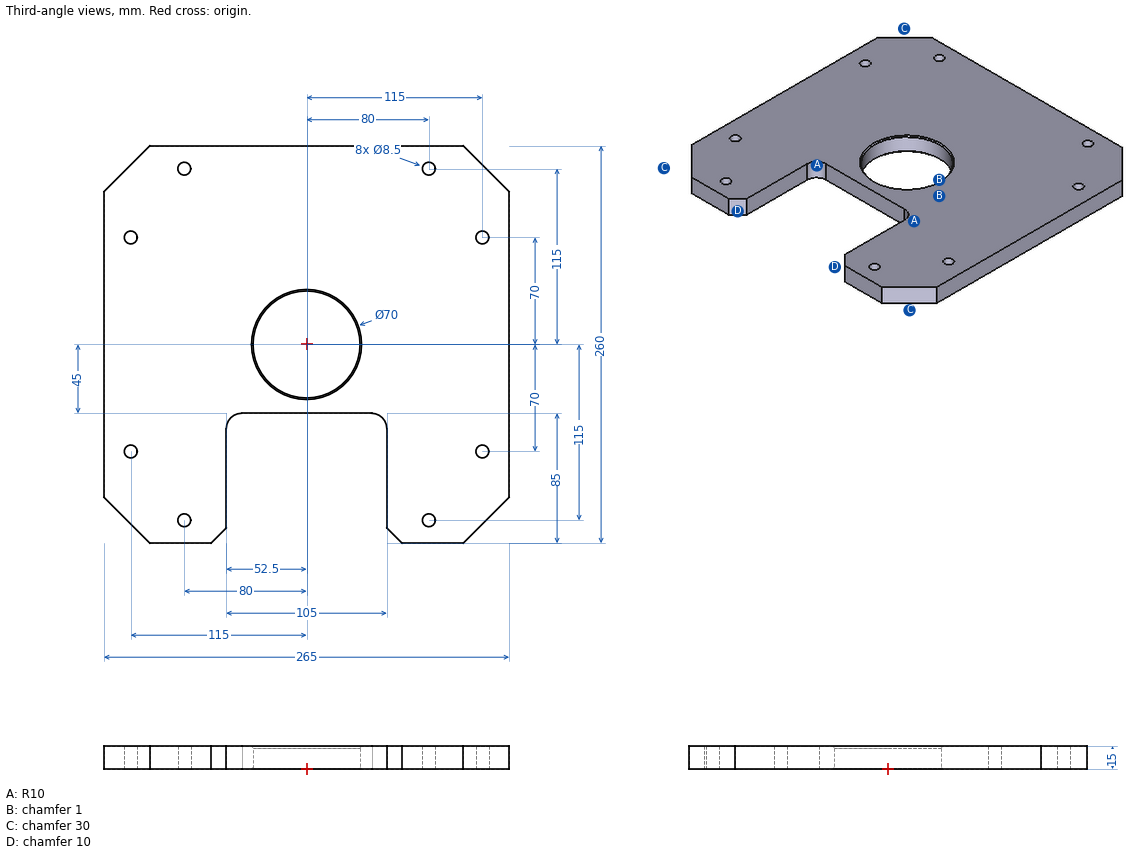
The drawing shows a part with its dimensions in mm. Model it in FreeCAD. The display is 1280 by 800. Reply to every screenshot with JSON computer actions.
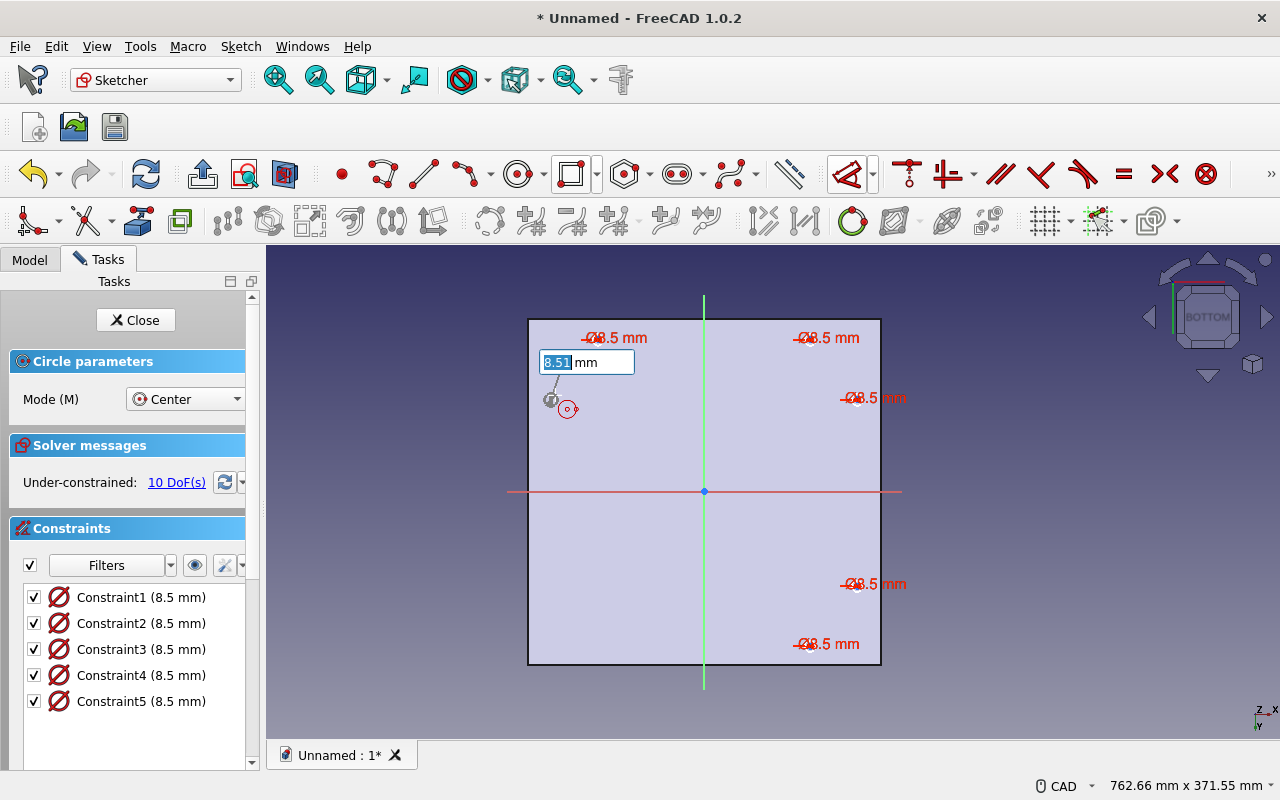
{"action": "type", "text": "8.5"}
{"action": "key", "text": "Return"}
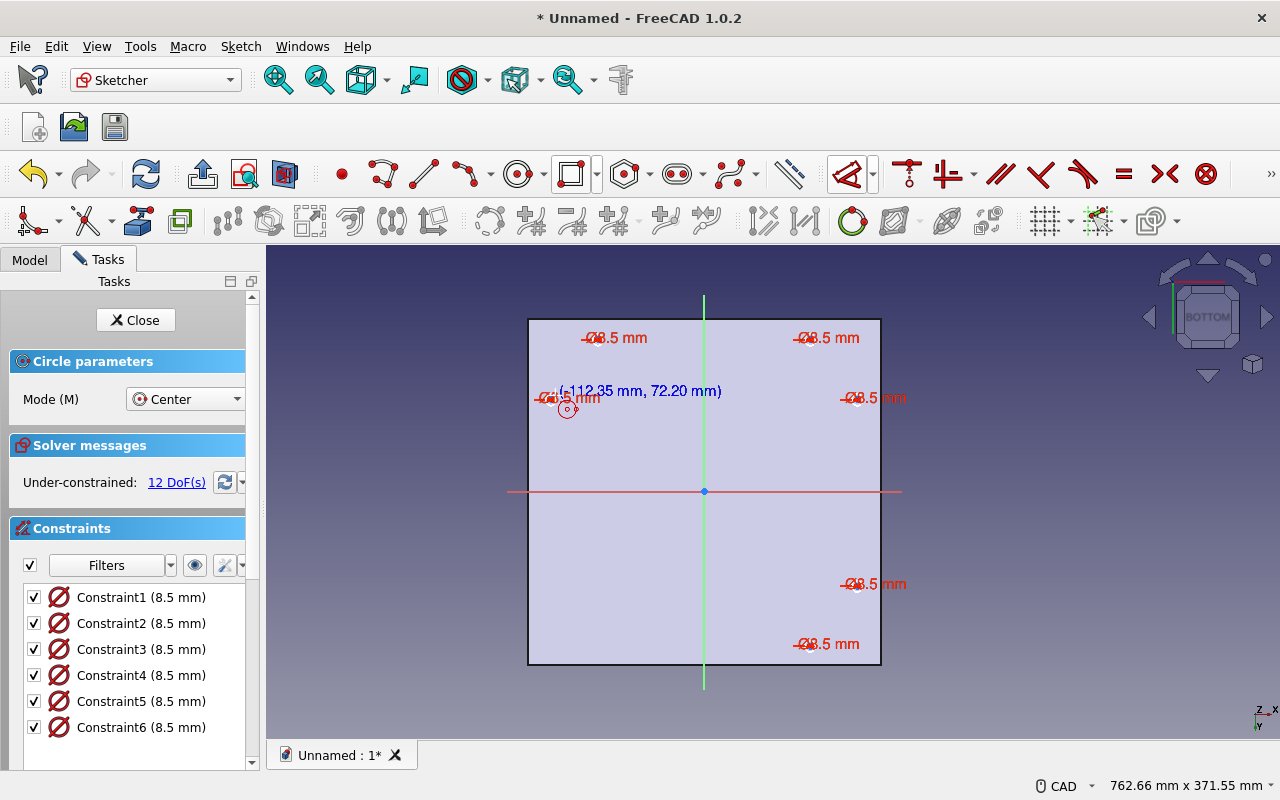
{"action": "scroll", "coordinate": [551, 585], "scroll_direction": "up", "scroll_amount": 7}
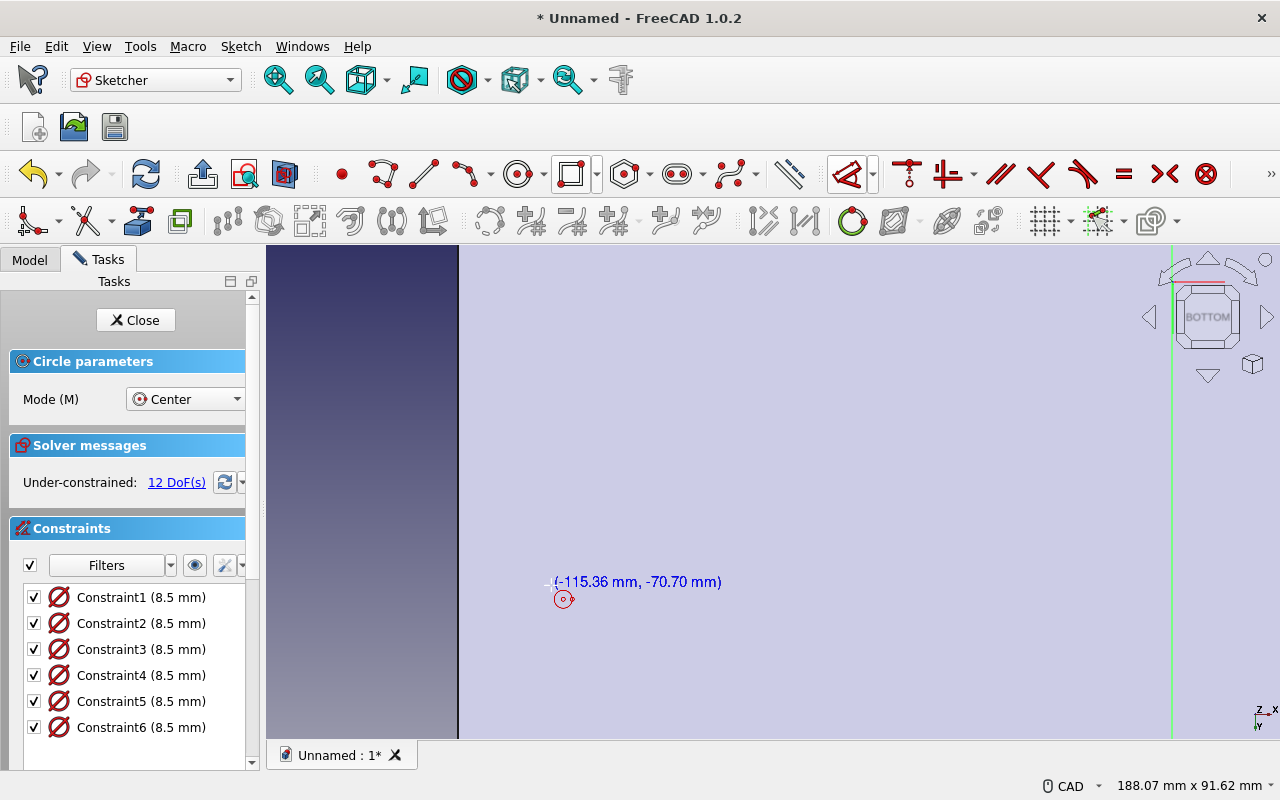
{"action": "scroll", "coordinate": [551, 586], "scroll_direction": "down", "scroll_amount": 7}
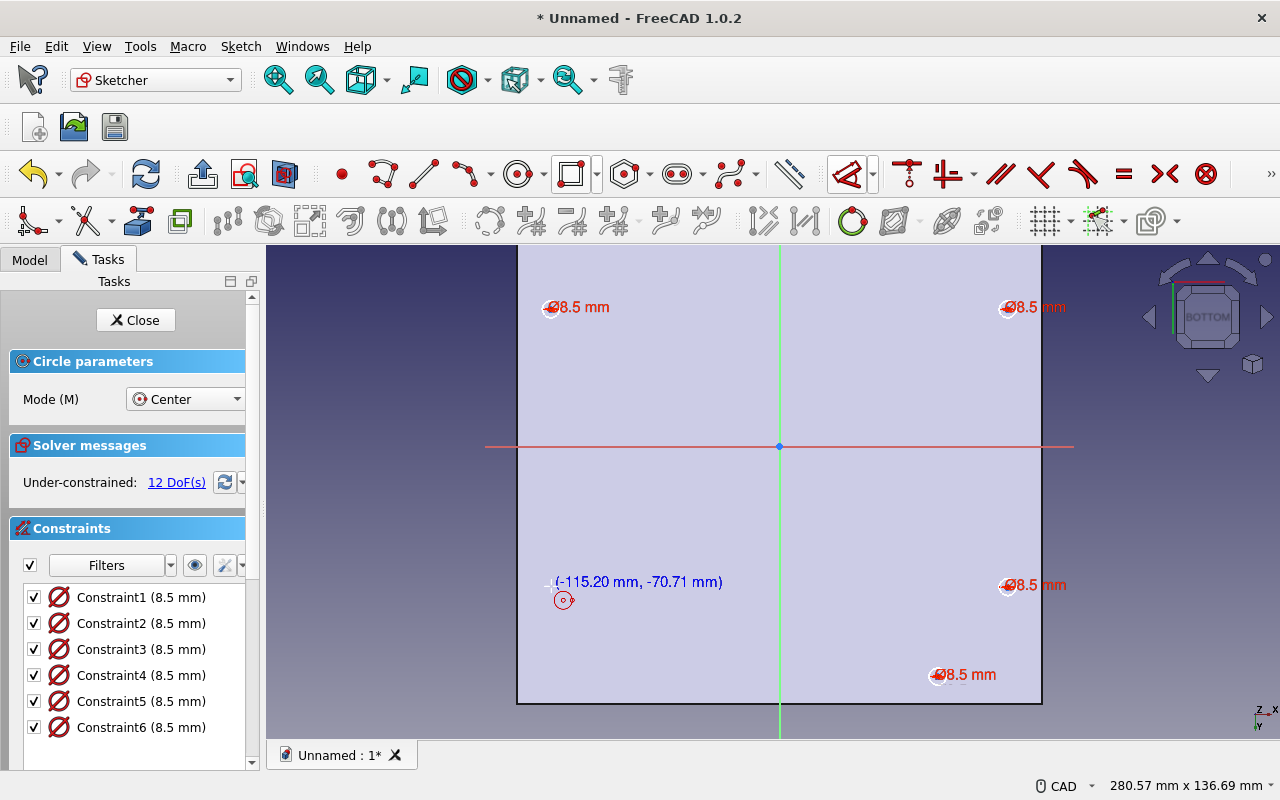
{"action": "left_click", "coordinate": [551, 586]}
{"action": "mouse_move", "coordinate": [555, 582]}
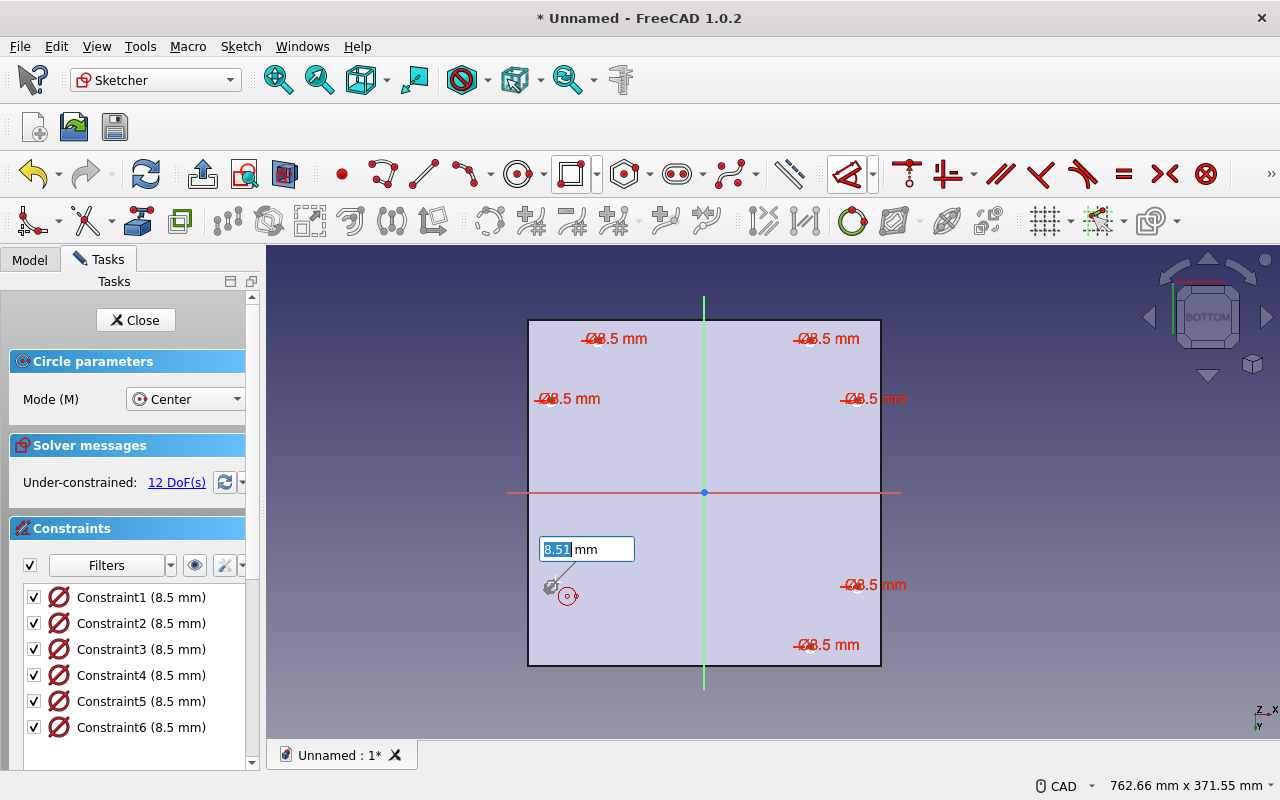
{"action": "type", "text": "8.5"}
{"action": "key", "text": "Return"}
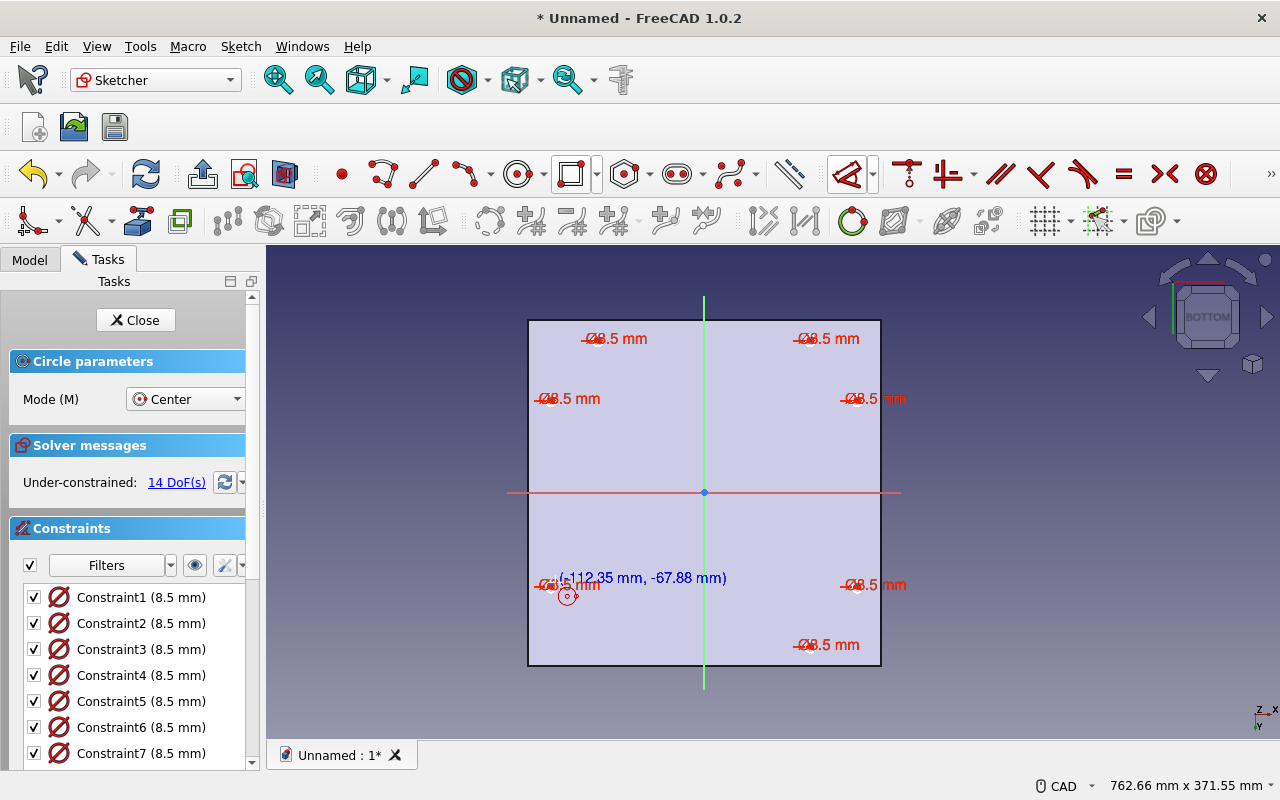
{"action": "scroll", "coordinate": [598, 646], "scroll_direction": "up", "scroll_amount": 7}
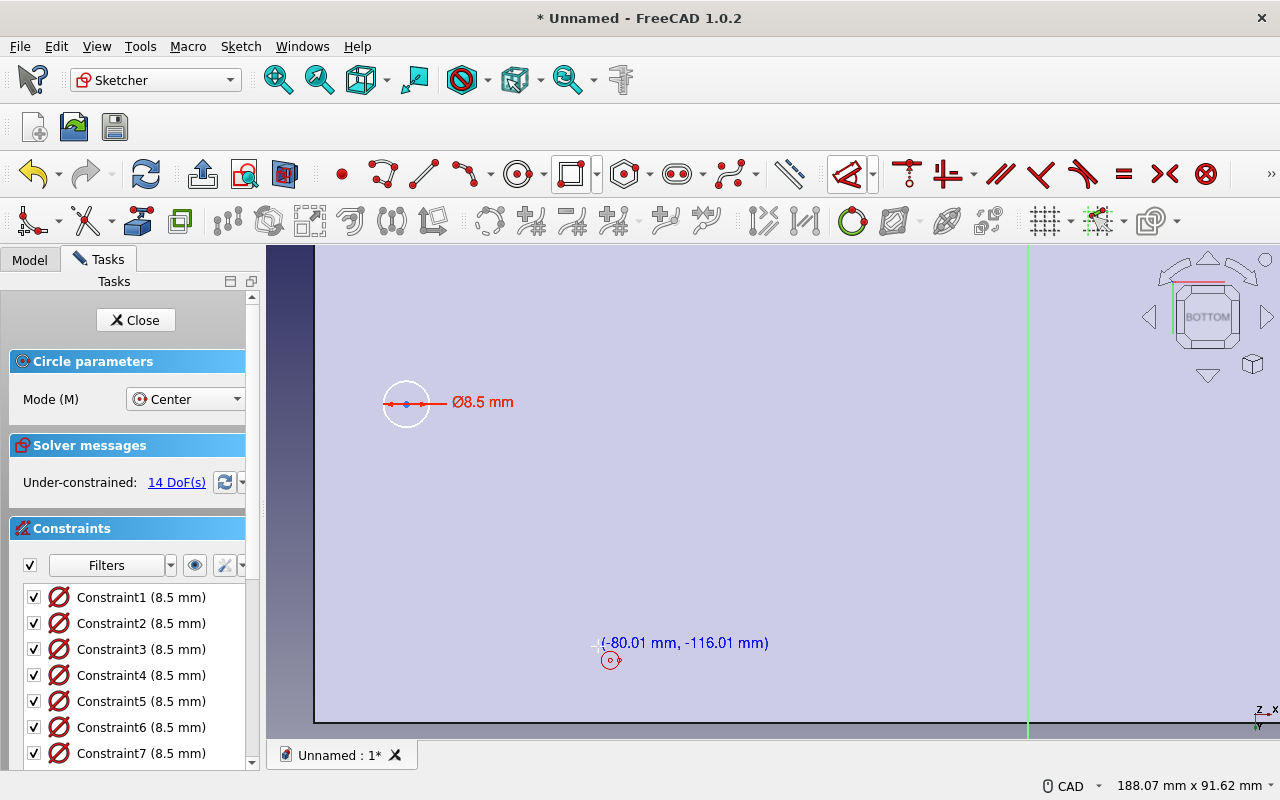
{"action": "scroll", "coordinate": [598, 646], "scroll_direction": "down", "scroll_amount": 7}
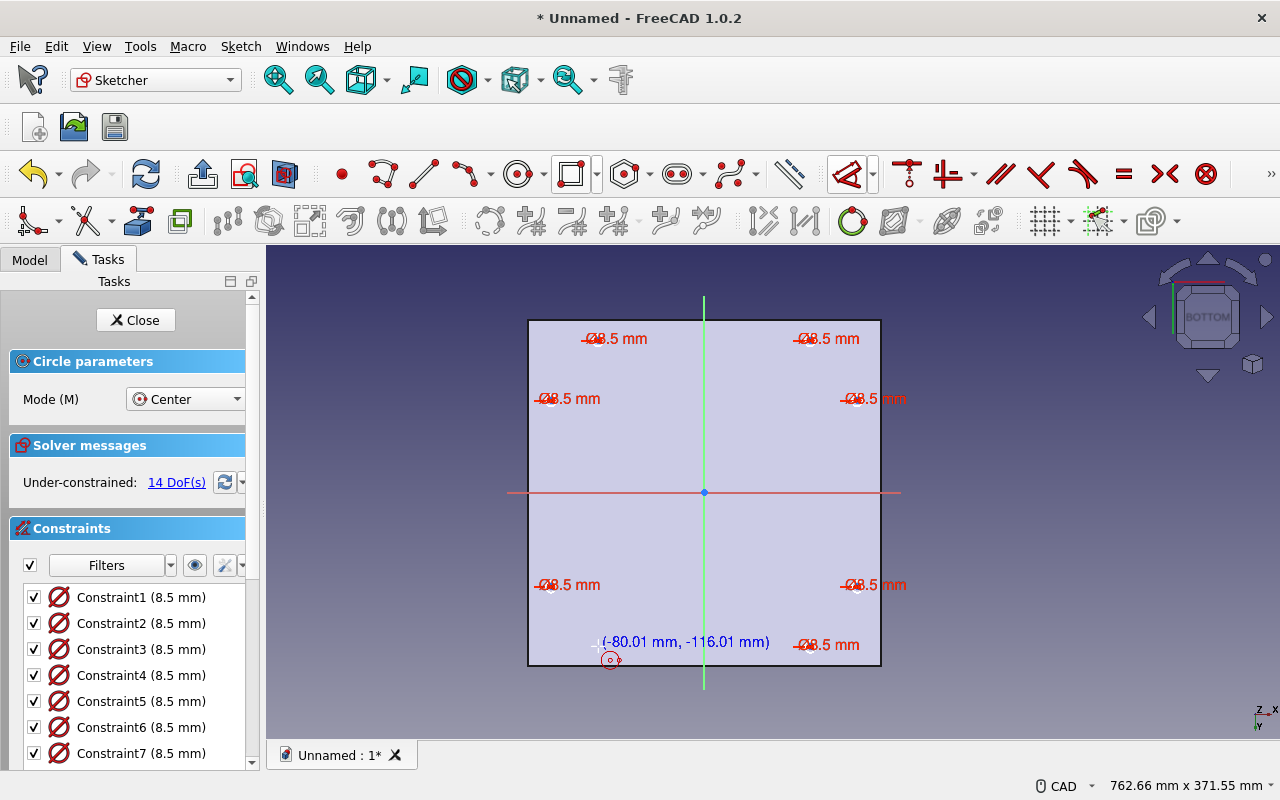
{"action": "left_click", "coordinate": [598, 646]}
{"action": "mouse_move", "coordinate": [602, 642]}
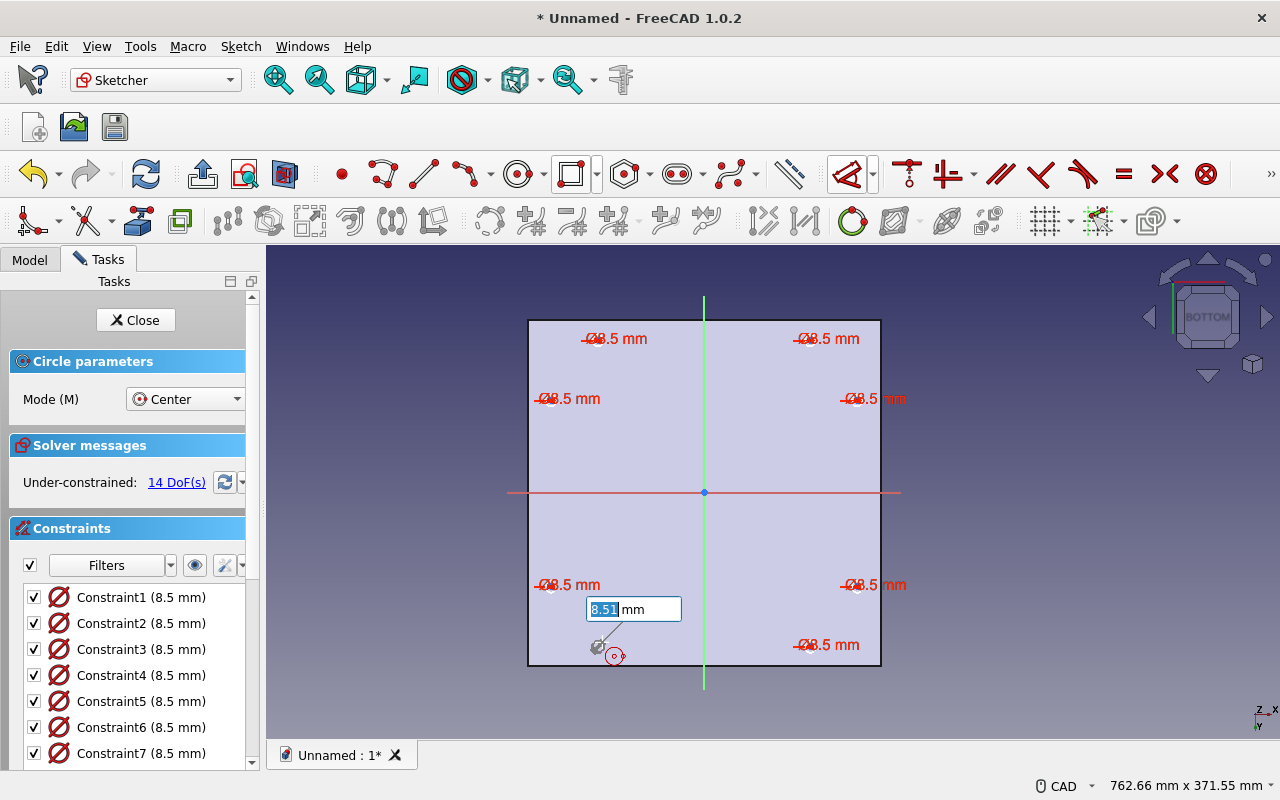
{"action": "type", "text": "8.5"}
{"action": "key", "text": "Return"}
{"action": "key", "text": "Escape"}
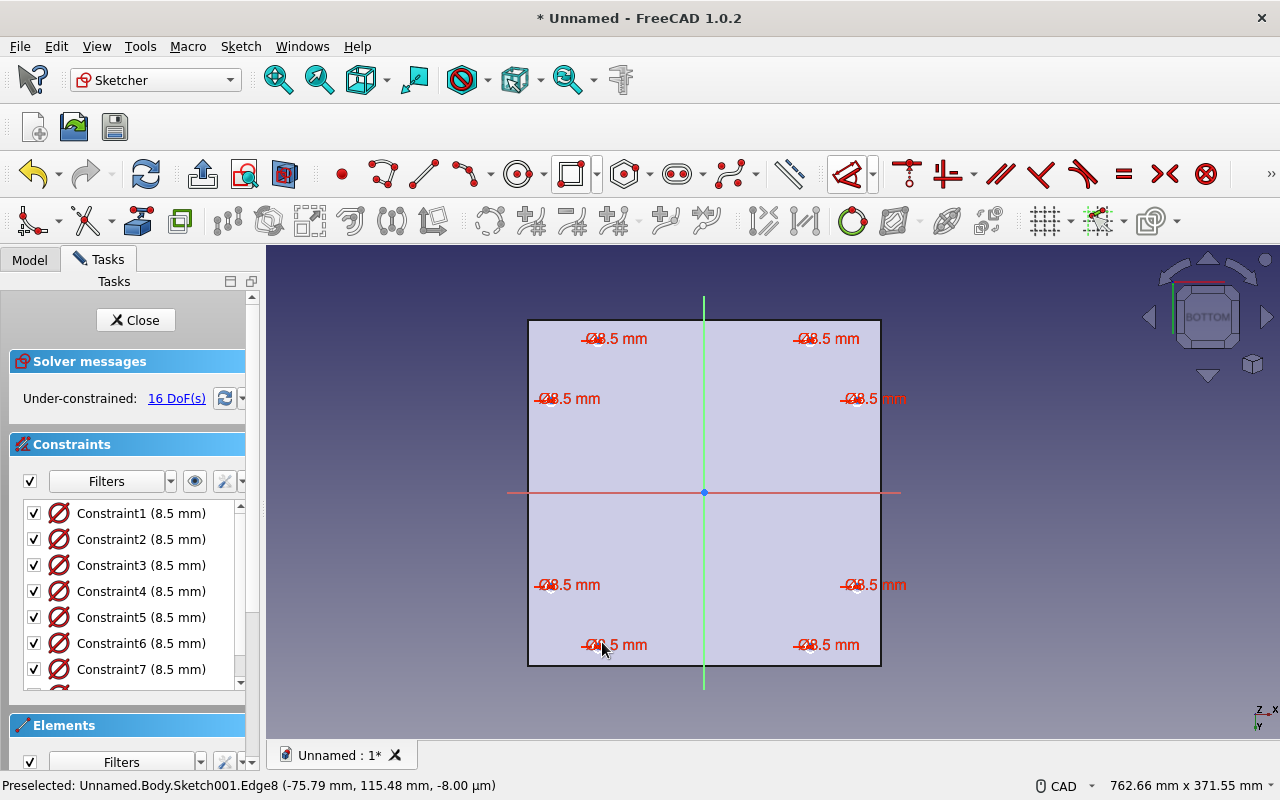
{"action": "left_click", "coordinate": [857, 587]}